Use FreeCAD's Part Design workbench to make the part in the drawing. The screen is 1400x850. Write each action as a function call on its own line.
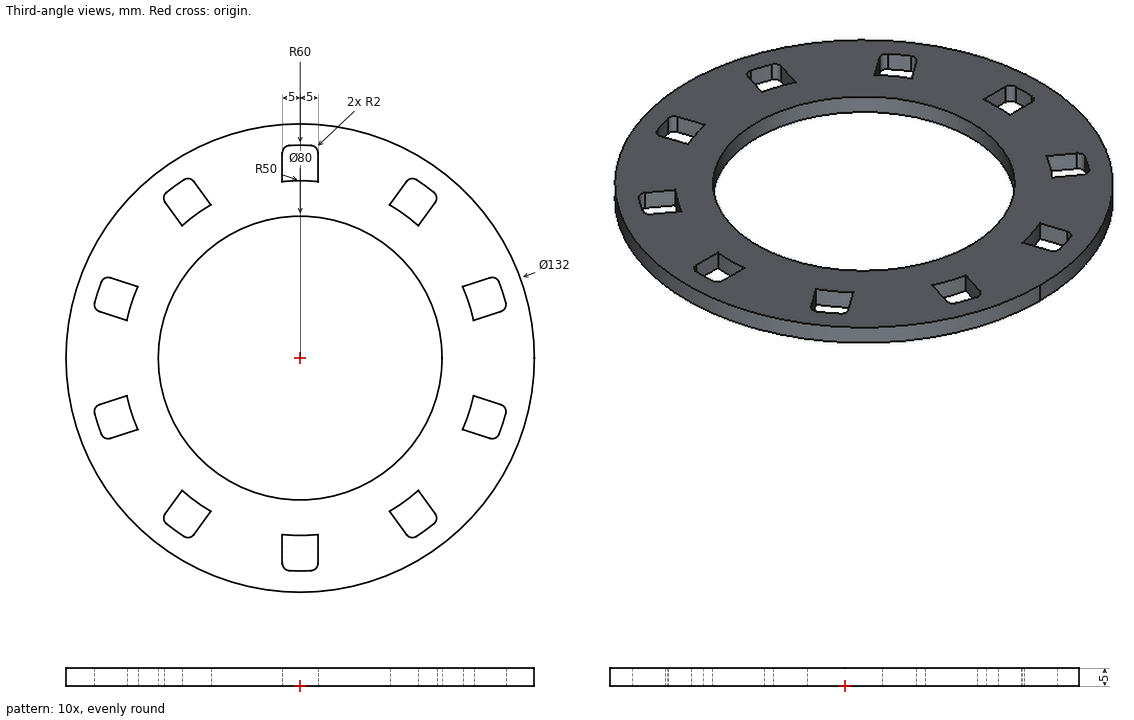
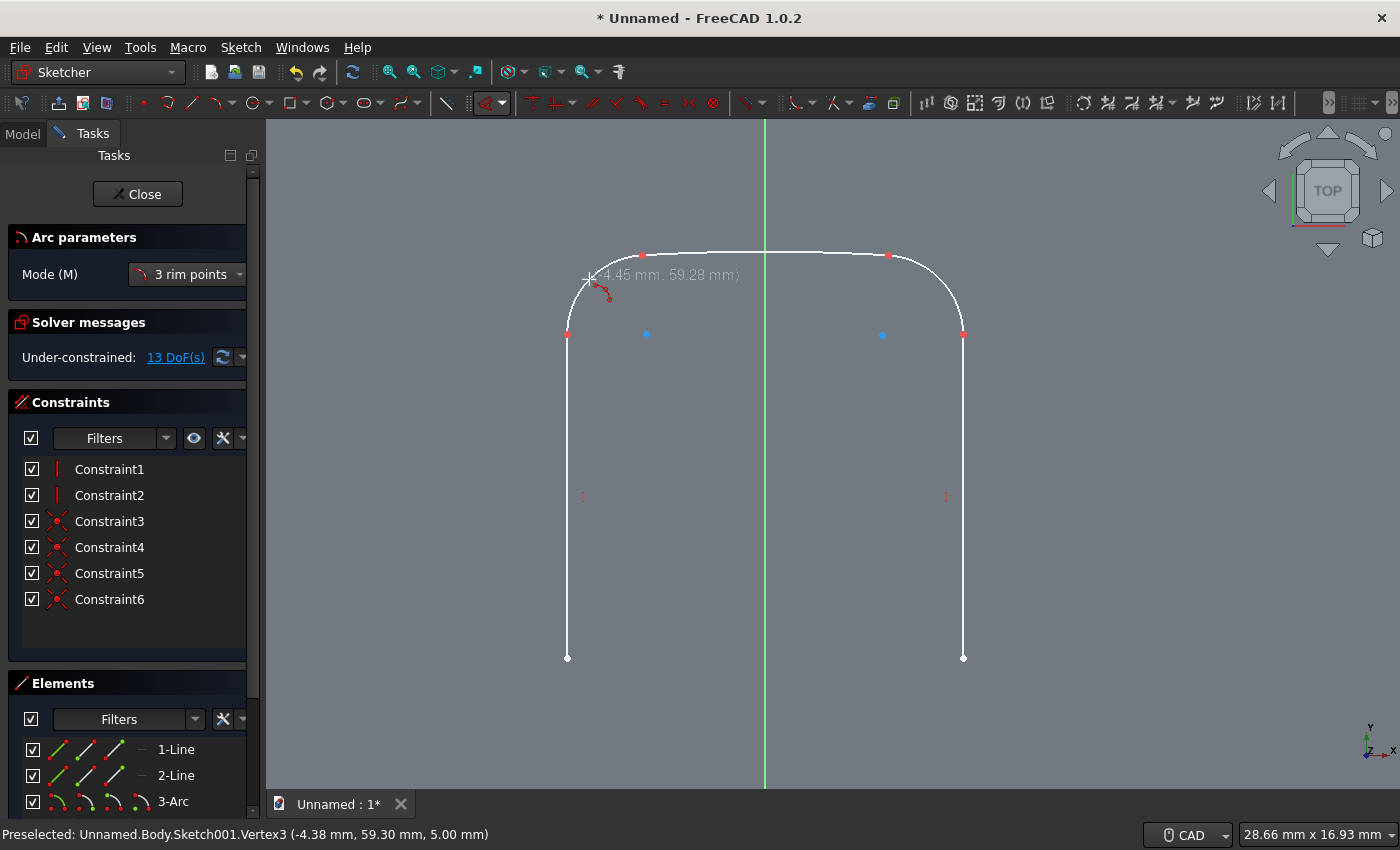
click(567, 658)
click(963, 658)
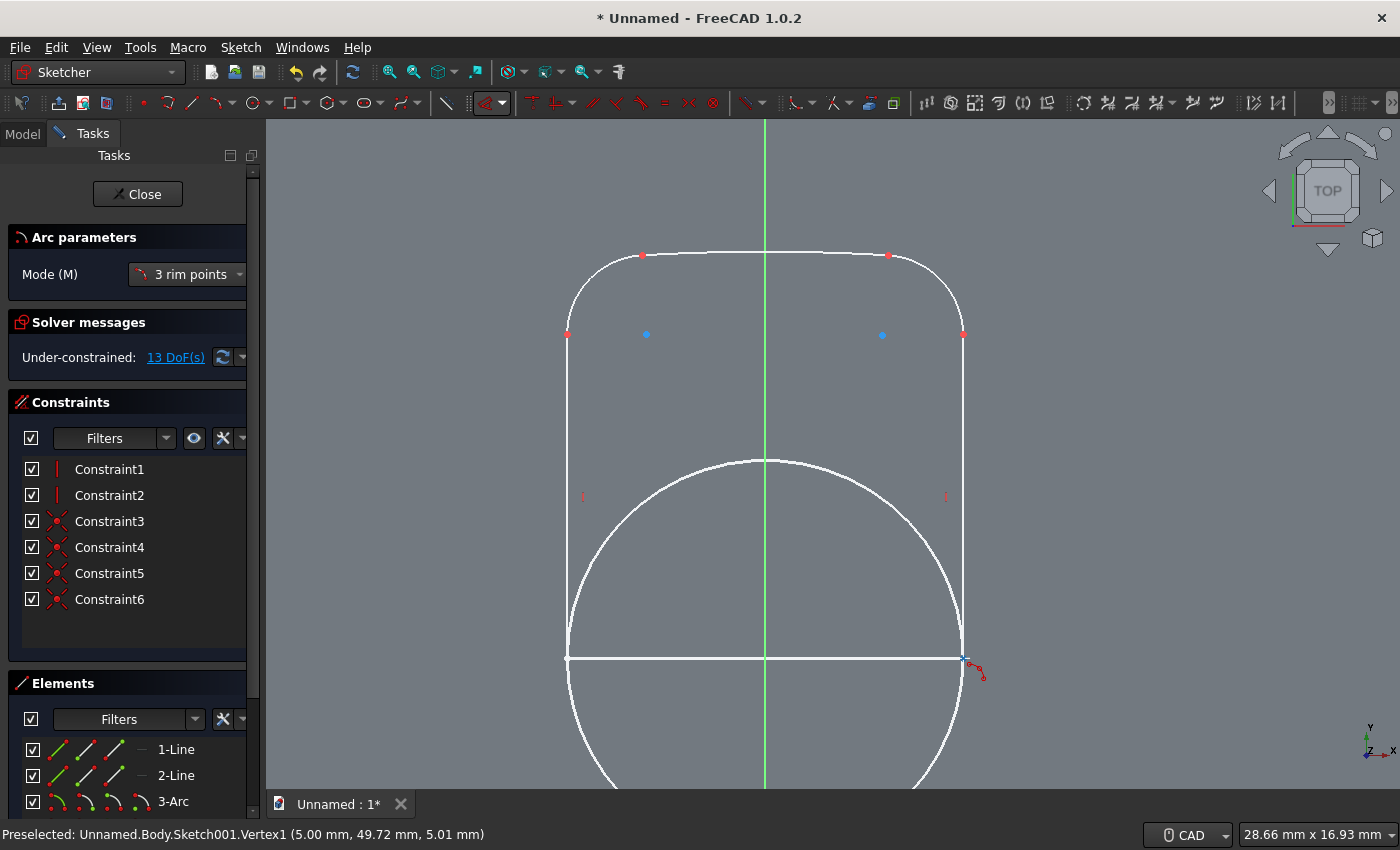
scroll(805, 648, up, 3)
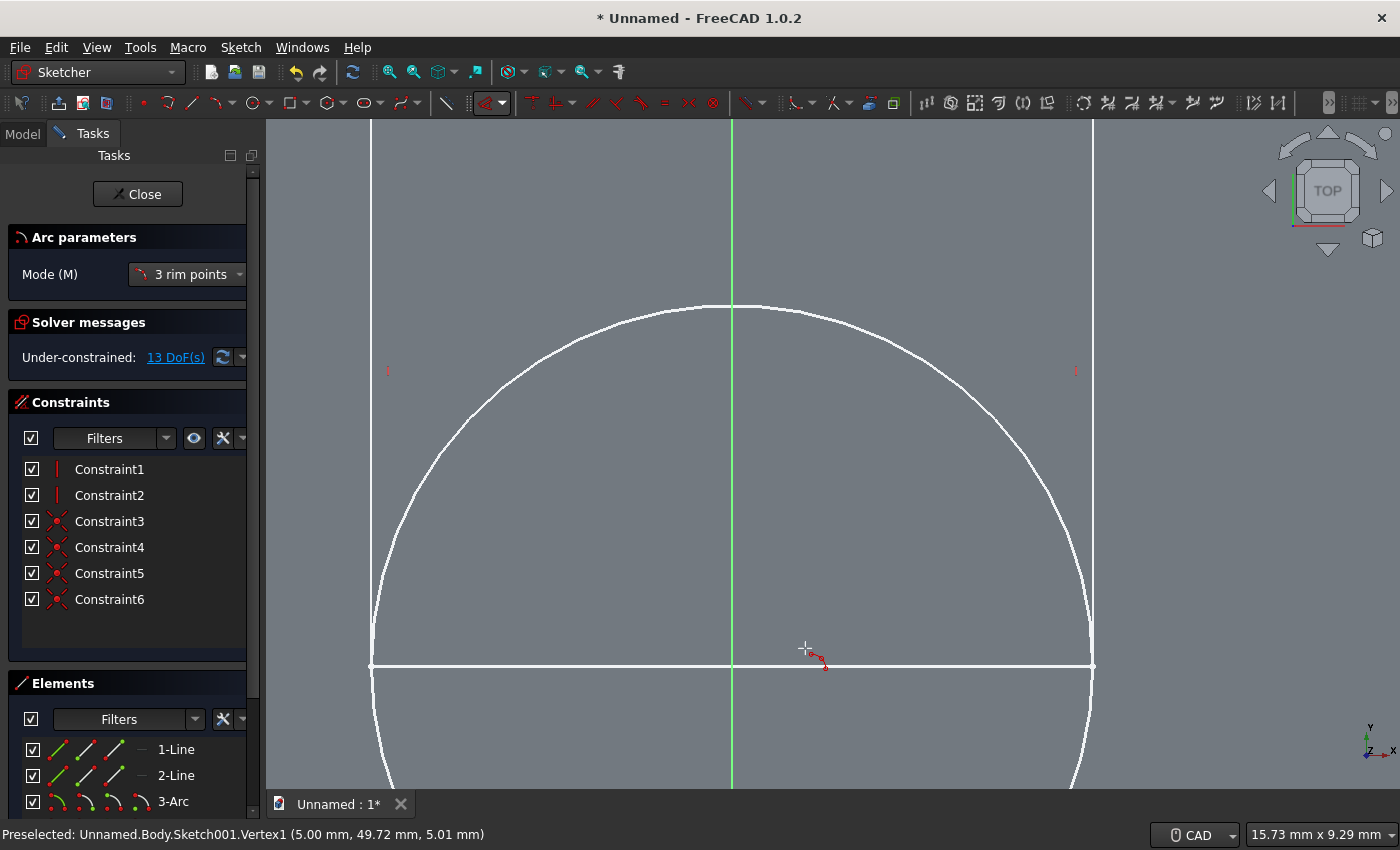
click(804, 647)
key(Escape)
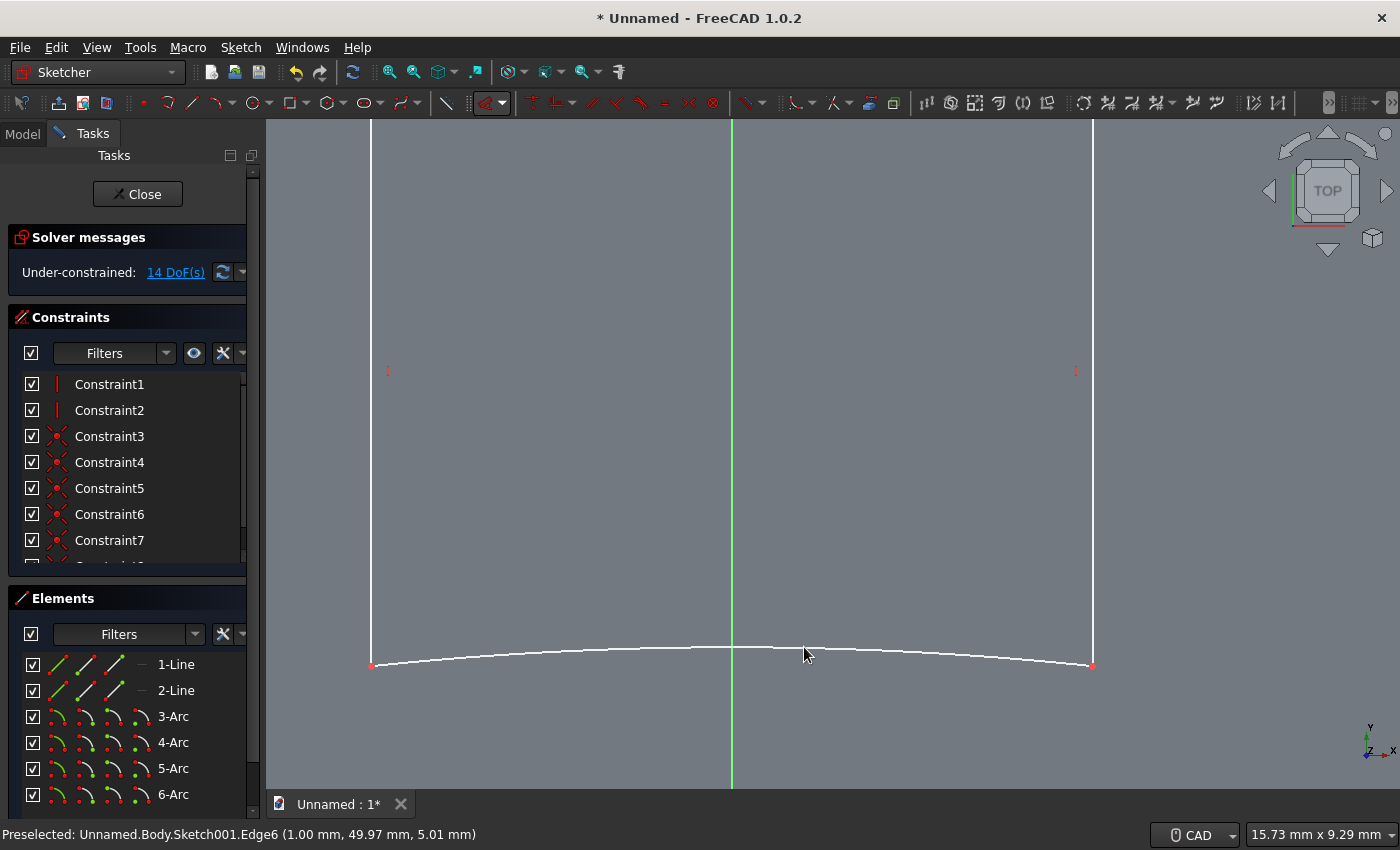
click(1093, 489)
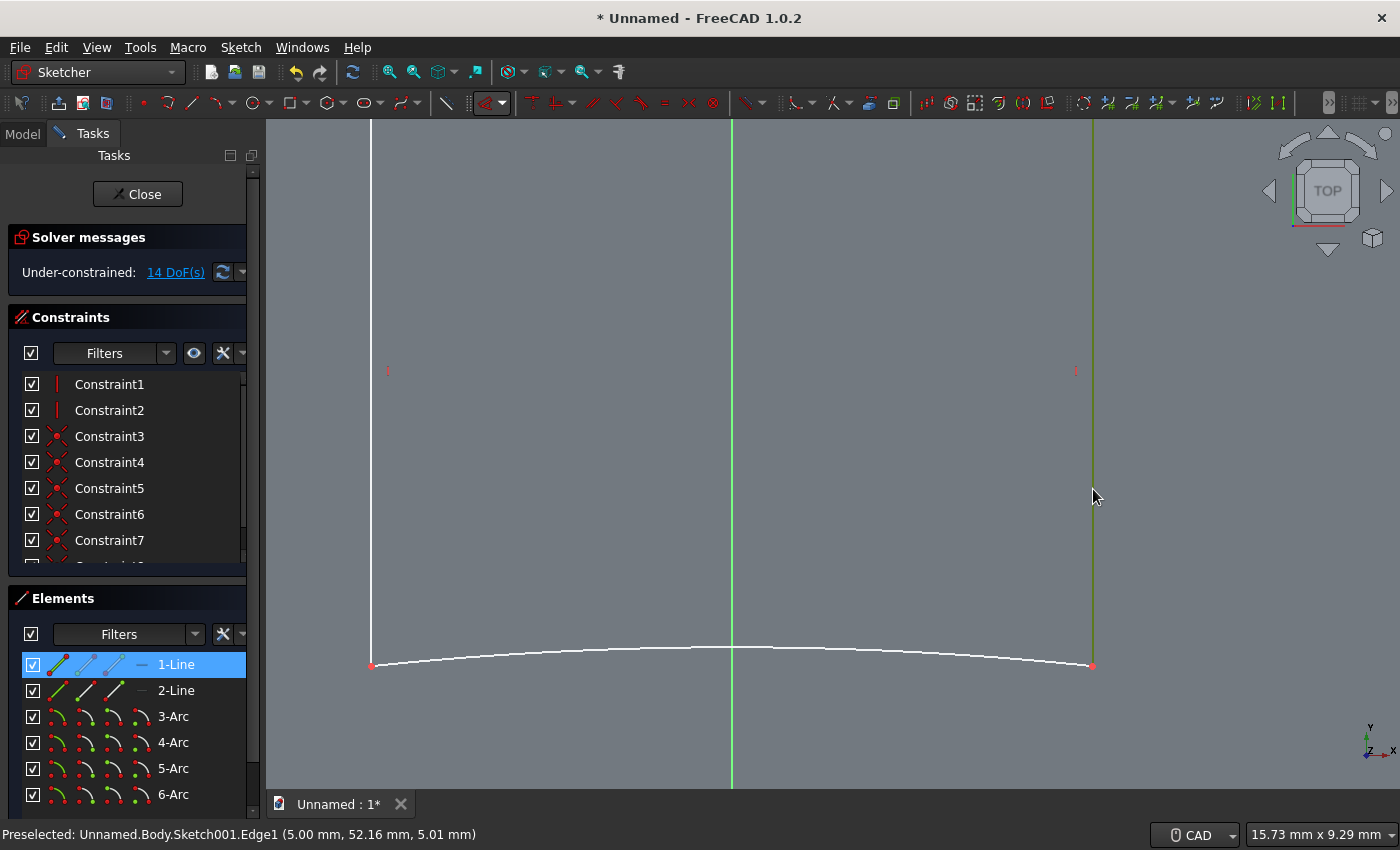
scroll(804, 648, down, 3)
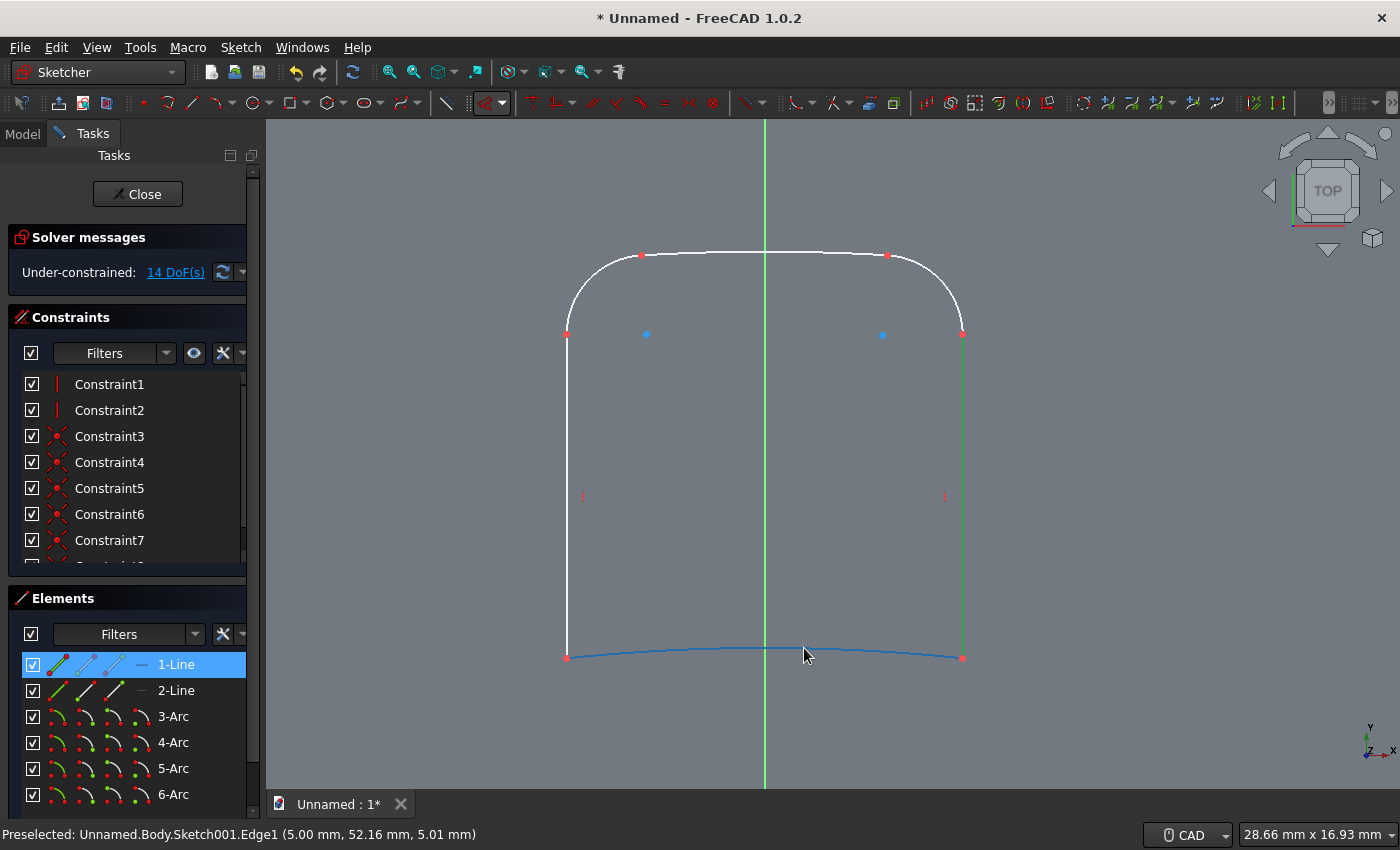
click(954, 300)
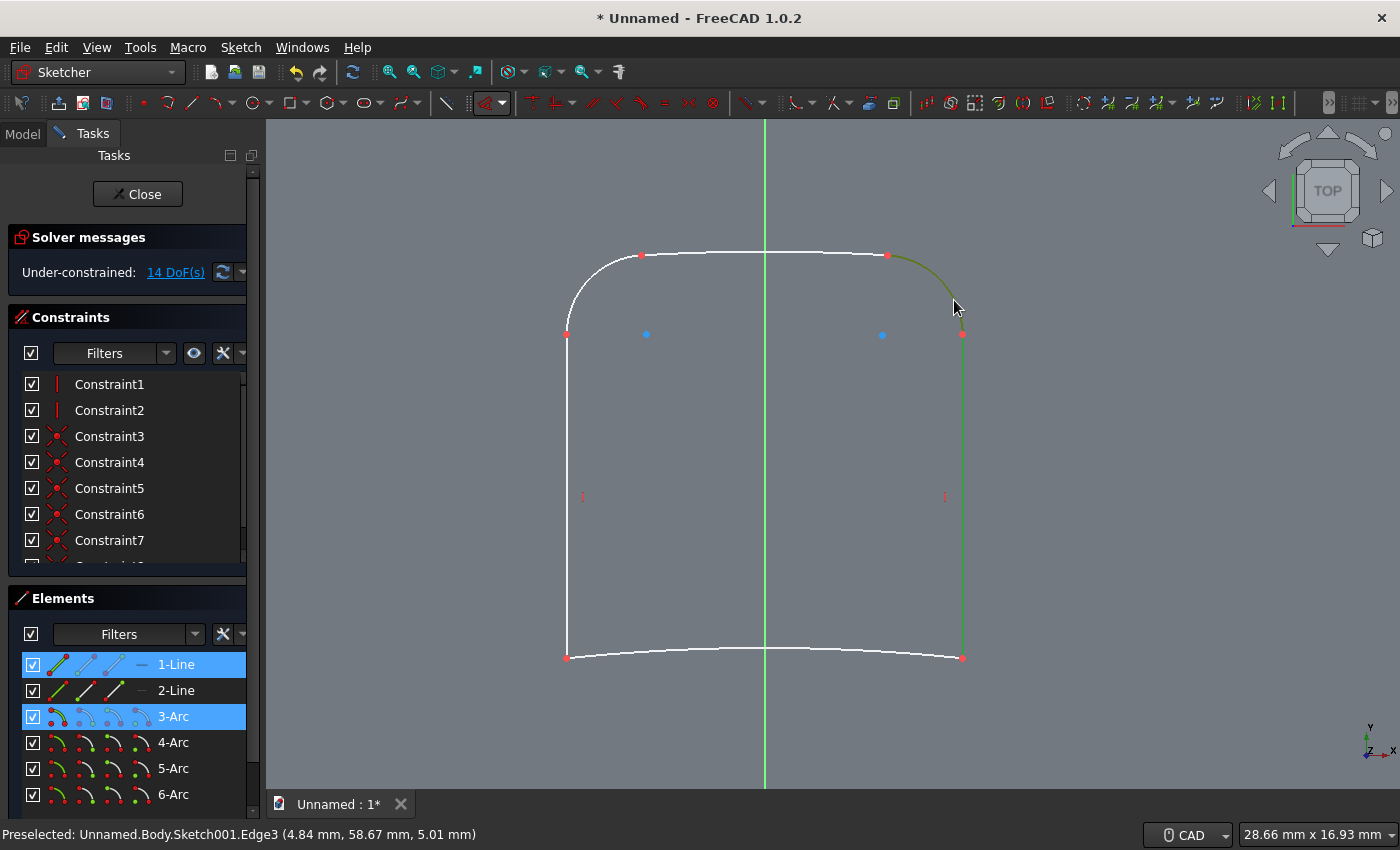
click(642, 104)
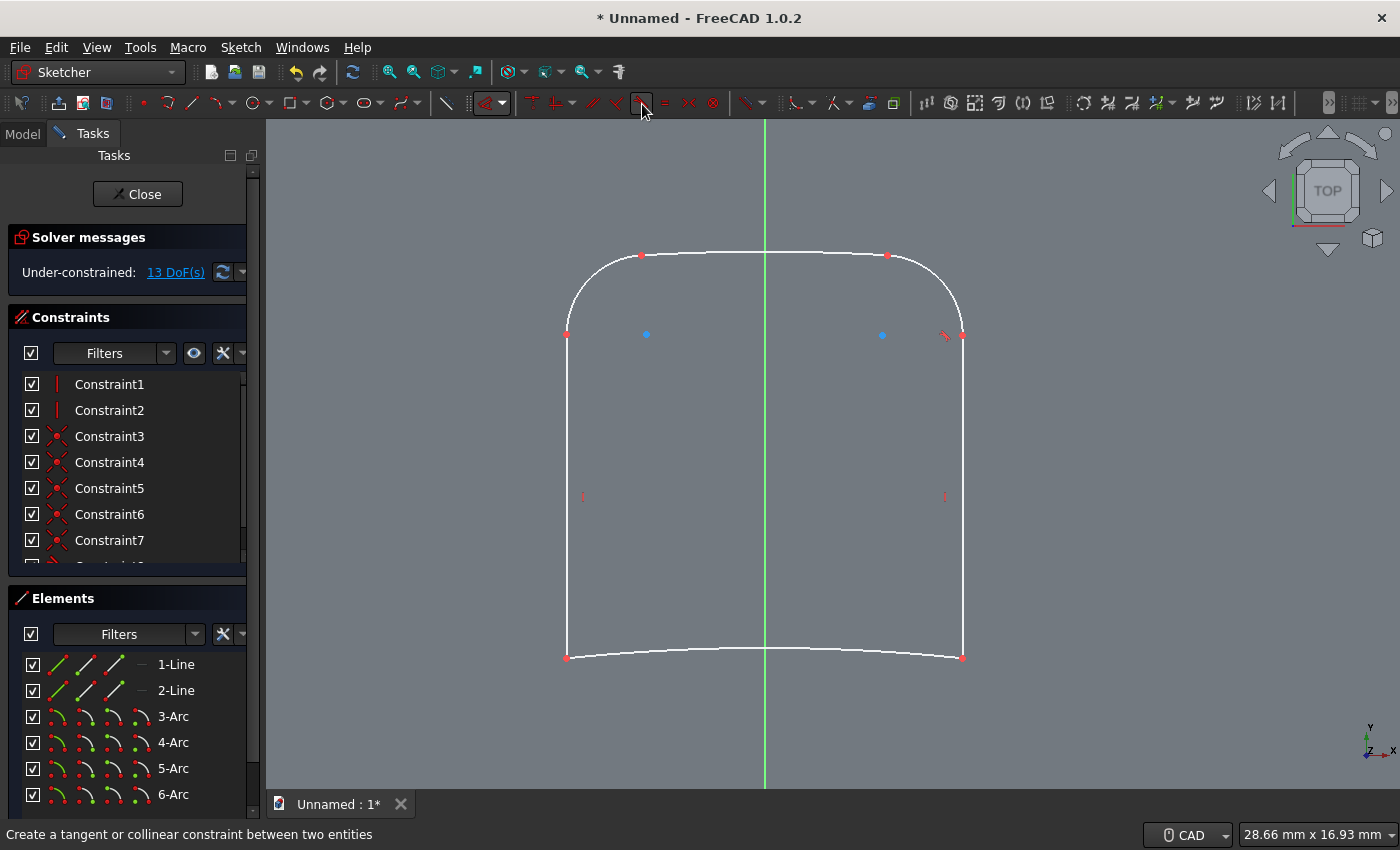
click(567, 432)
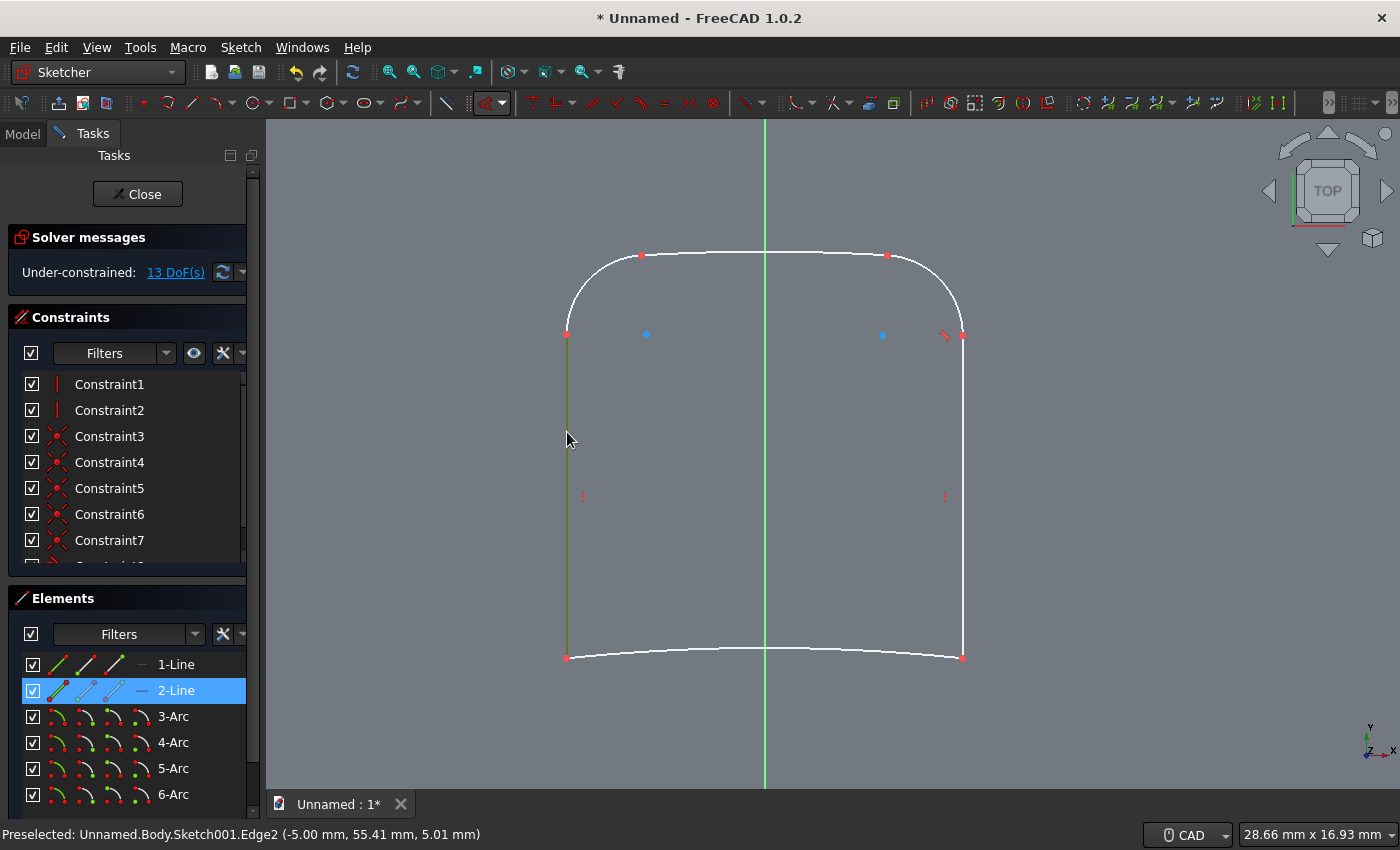
click(607, 265)